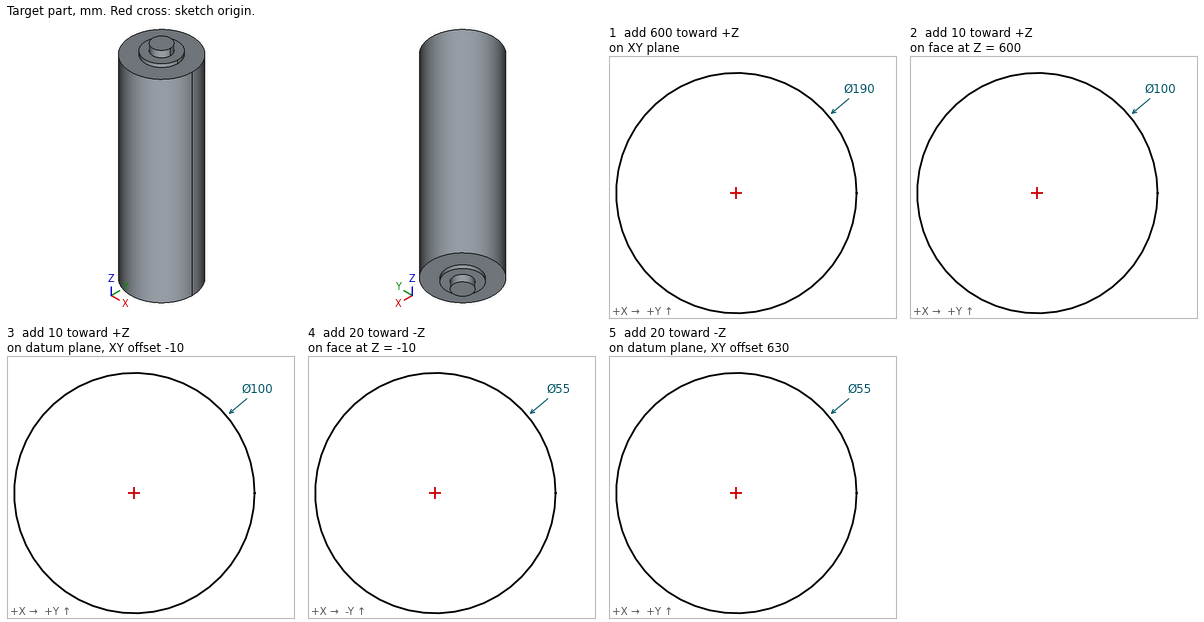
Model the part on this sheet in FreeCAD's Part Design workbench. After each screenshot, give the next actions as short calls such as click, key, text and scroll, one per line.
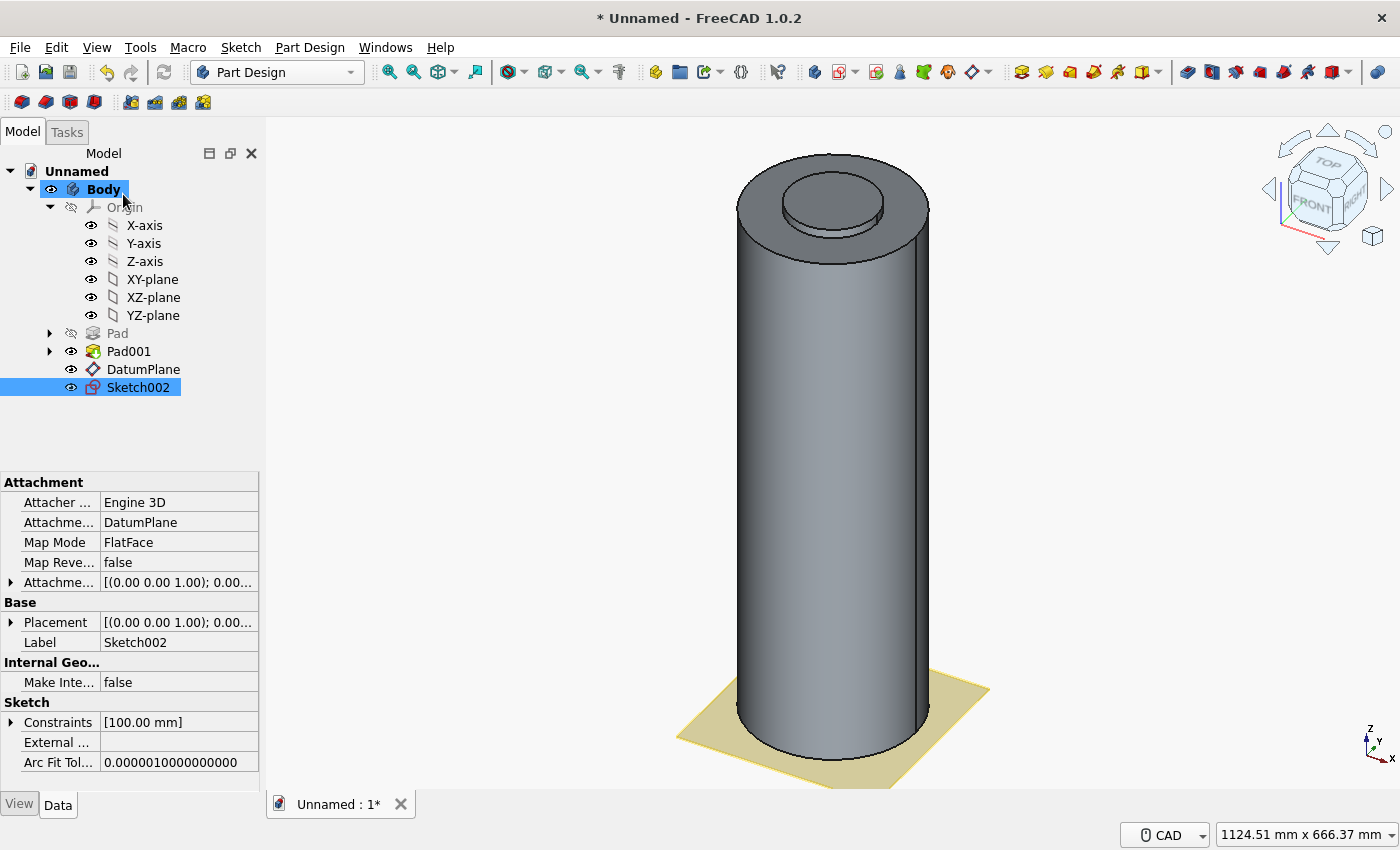
click(1022, 72)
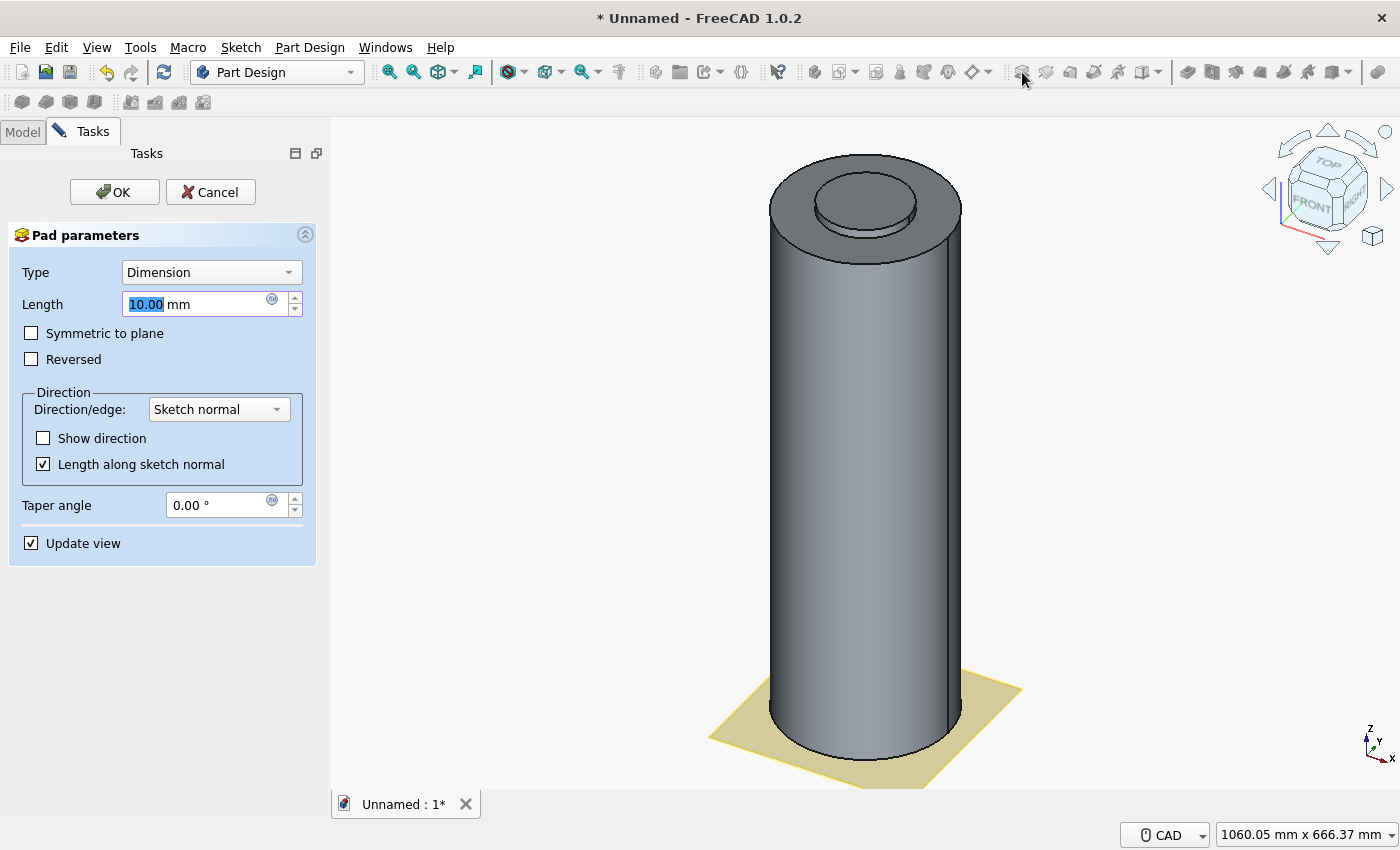
text(10)
key(Tab)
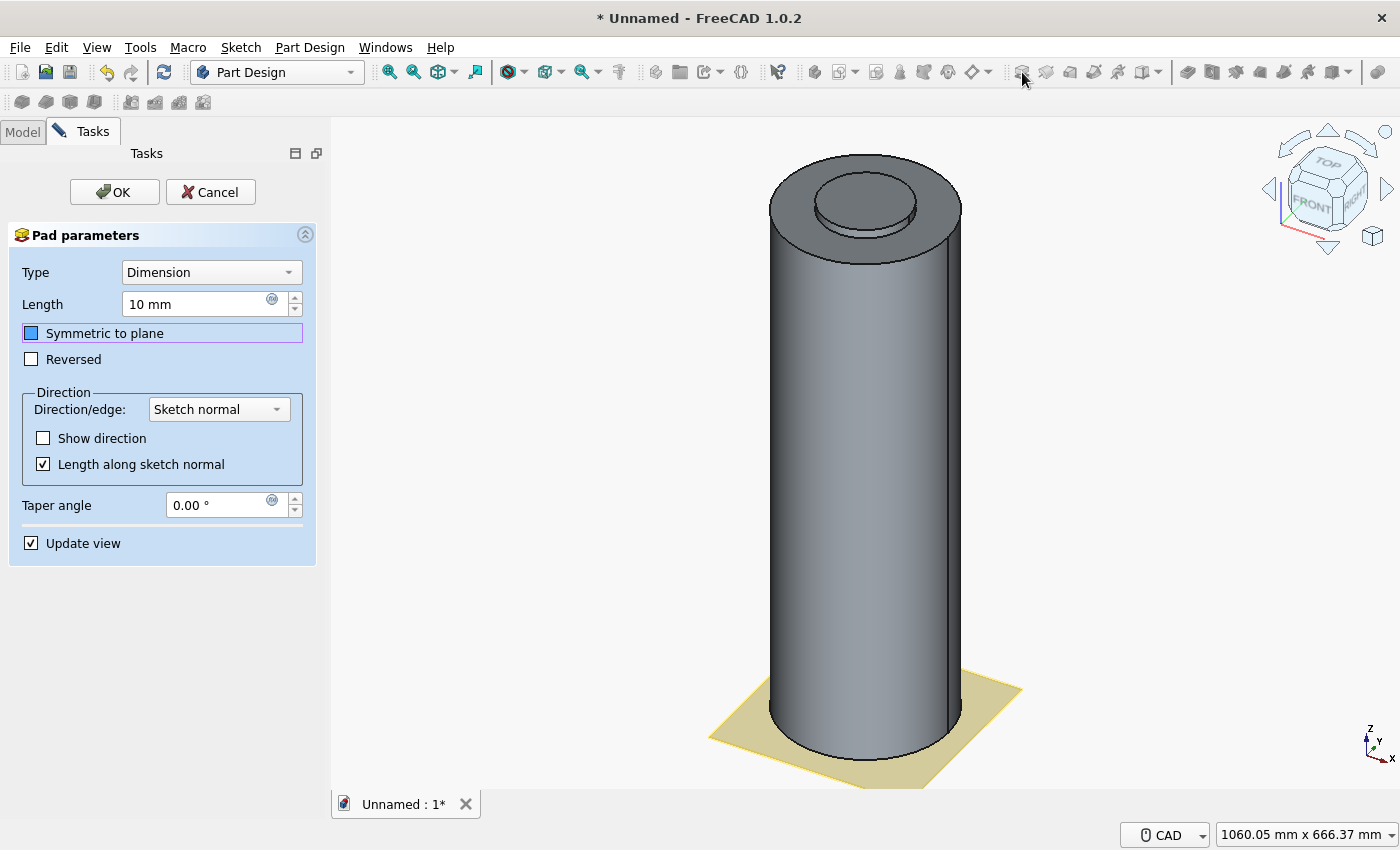
click(115, 192)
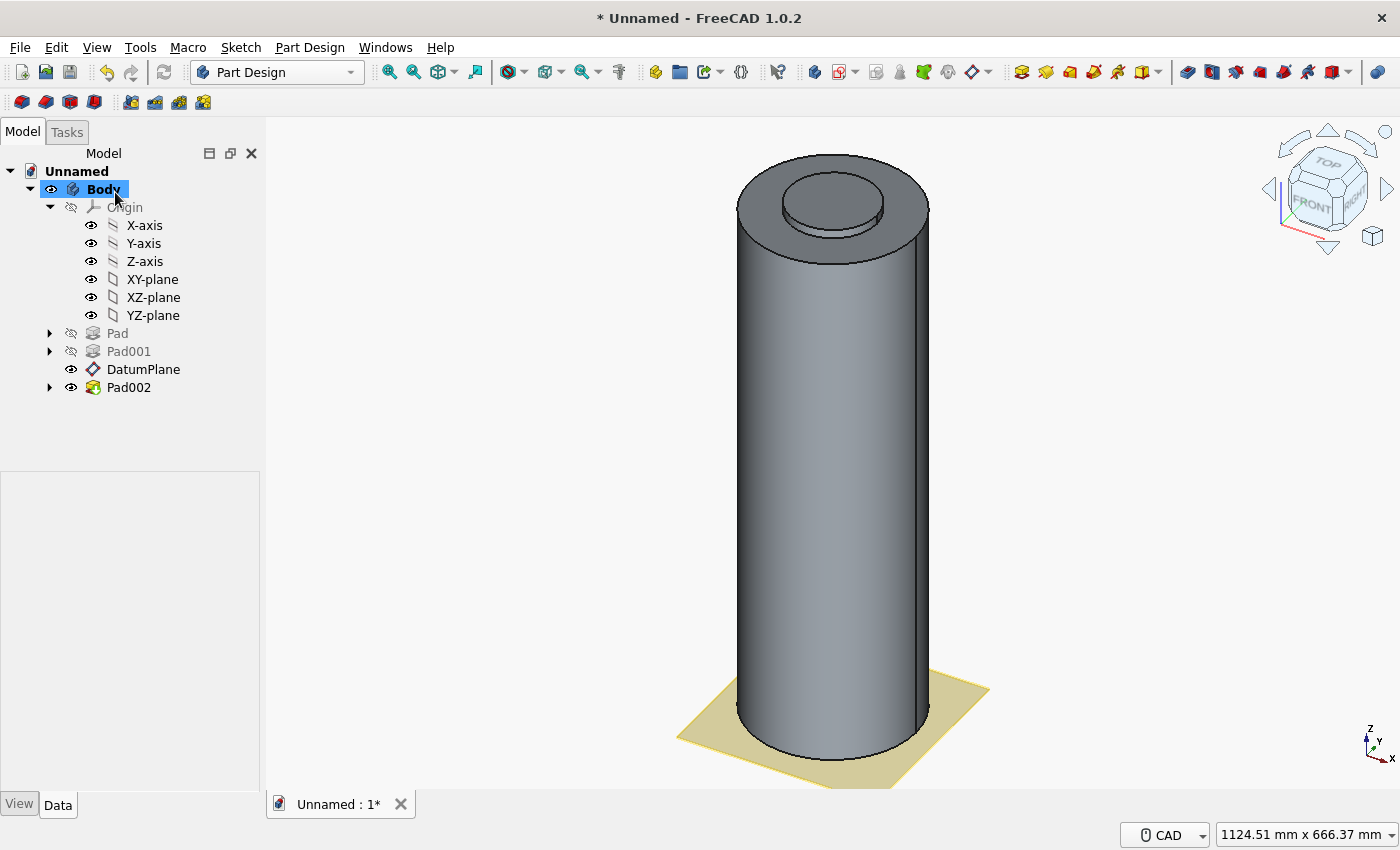
click(116, 369)
key(space)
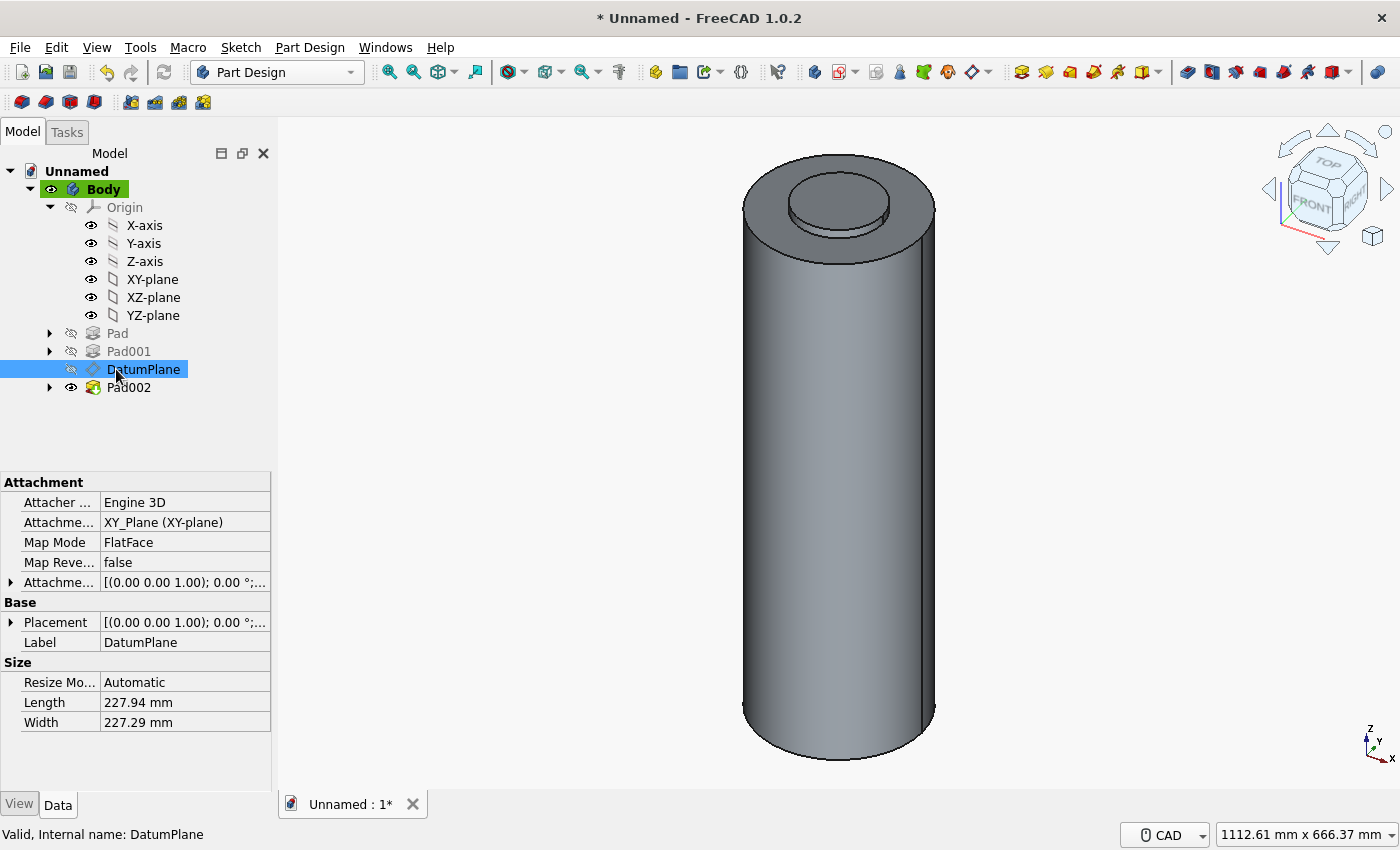
key(5)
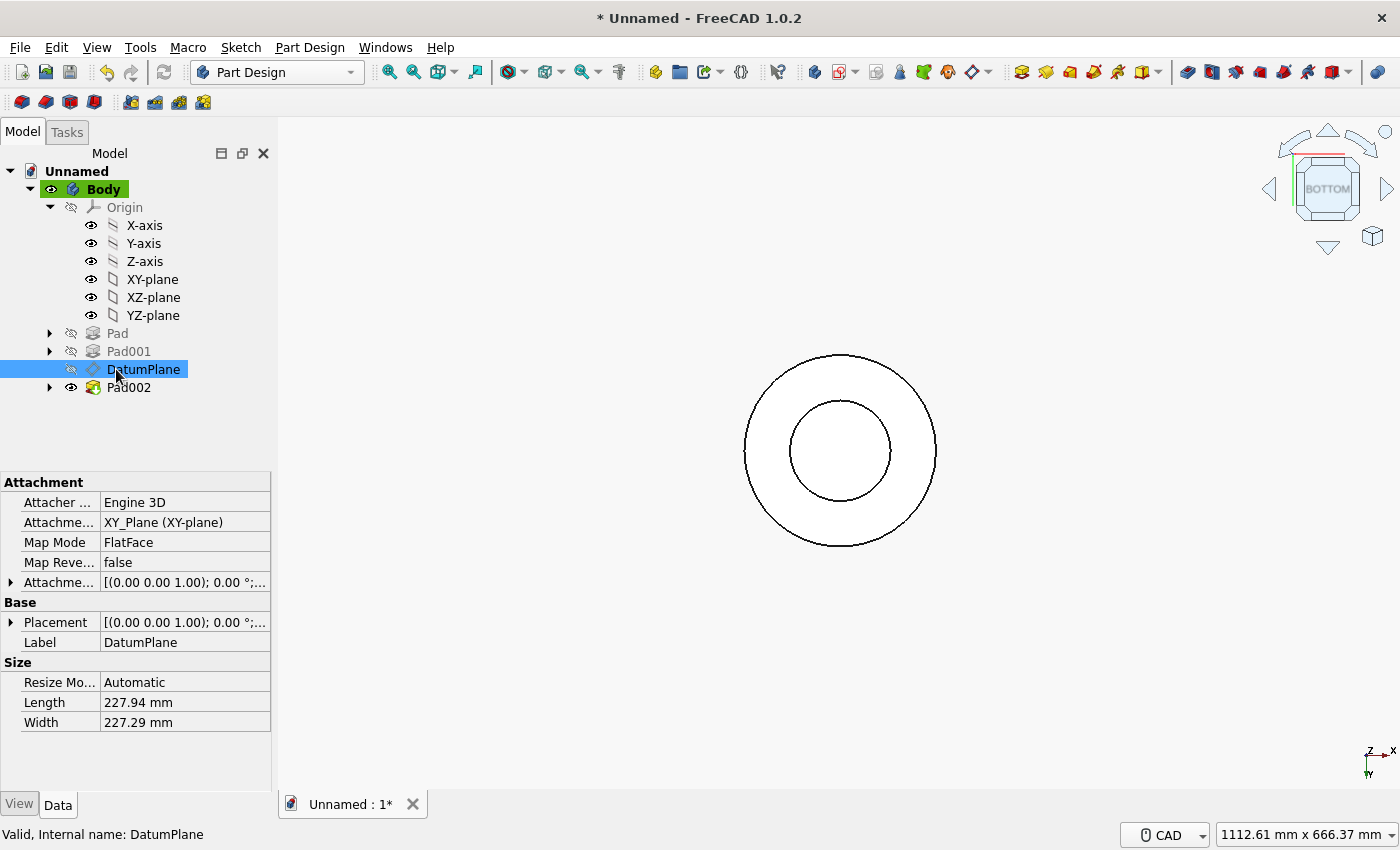
key(v)
key(f)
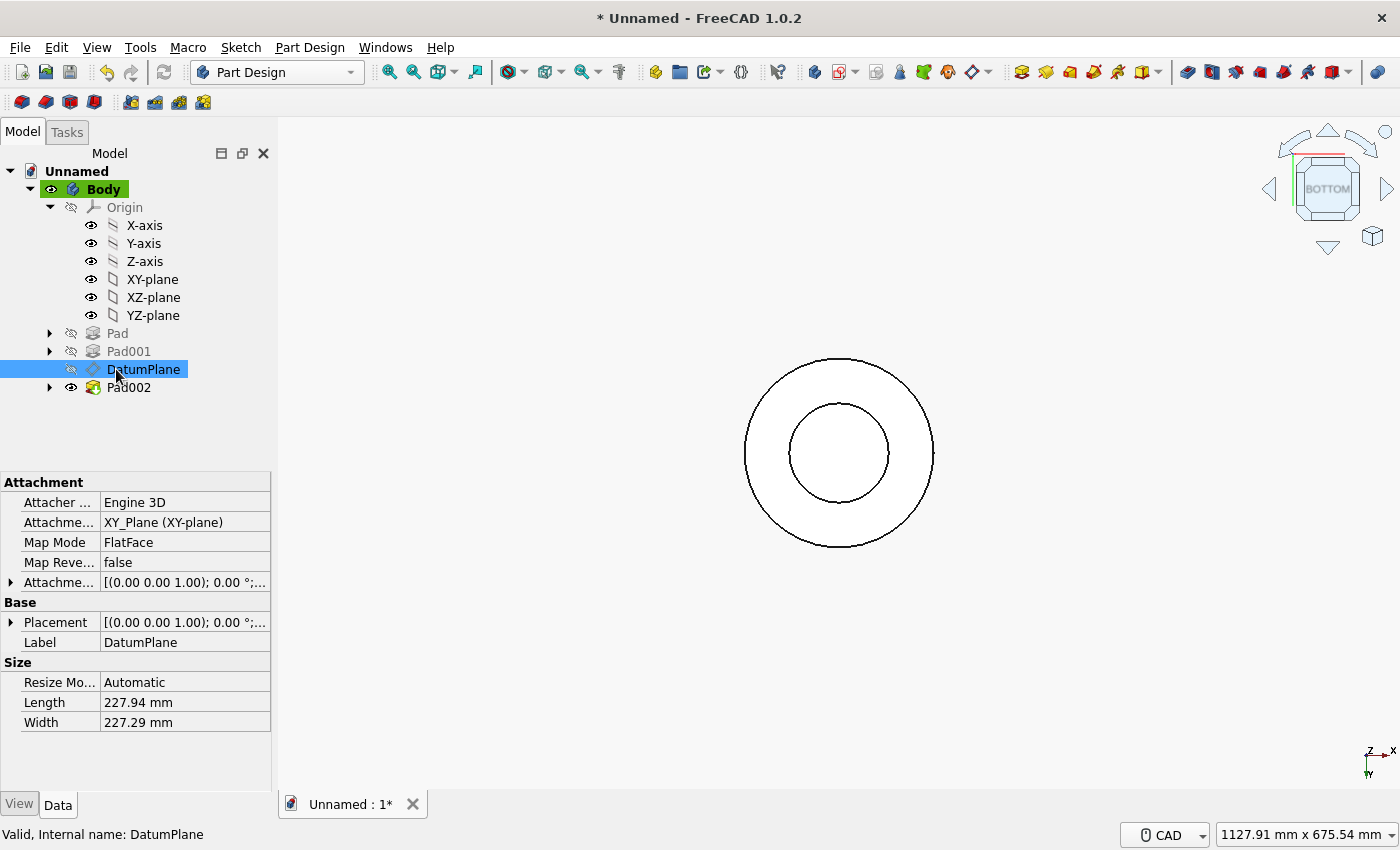
click(839, 452)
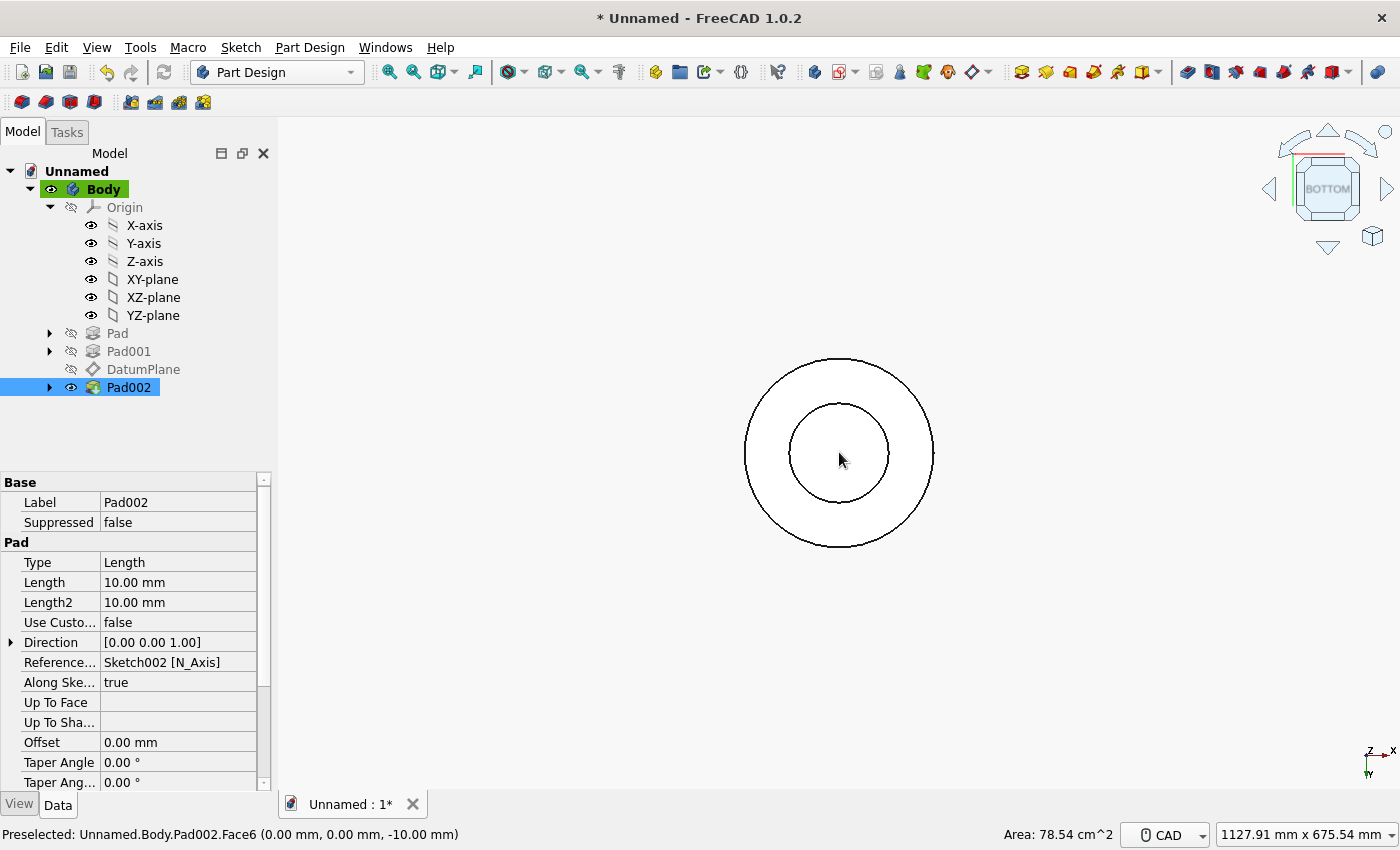
click(840, 72)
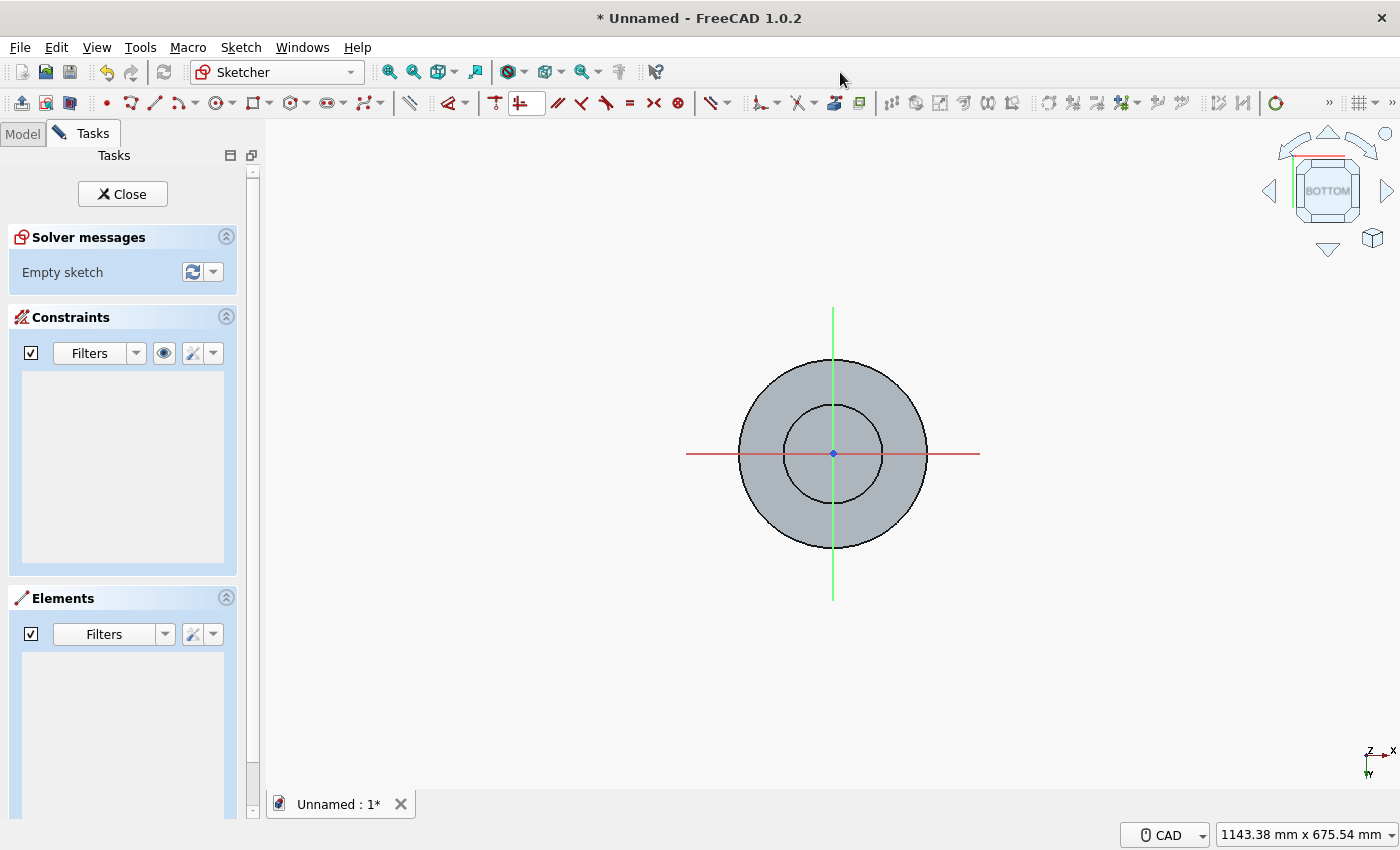
scroll(844, 454, up, 10)